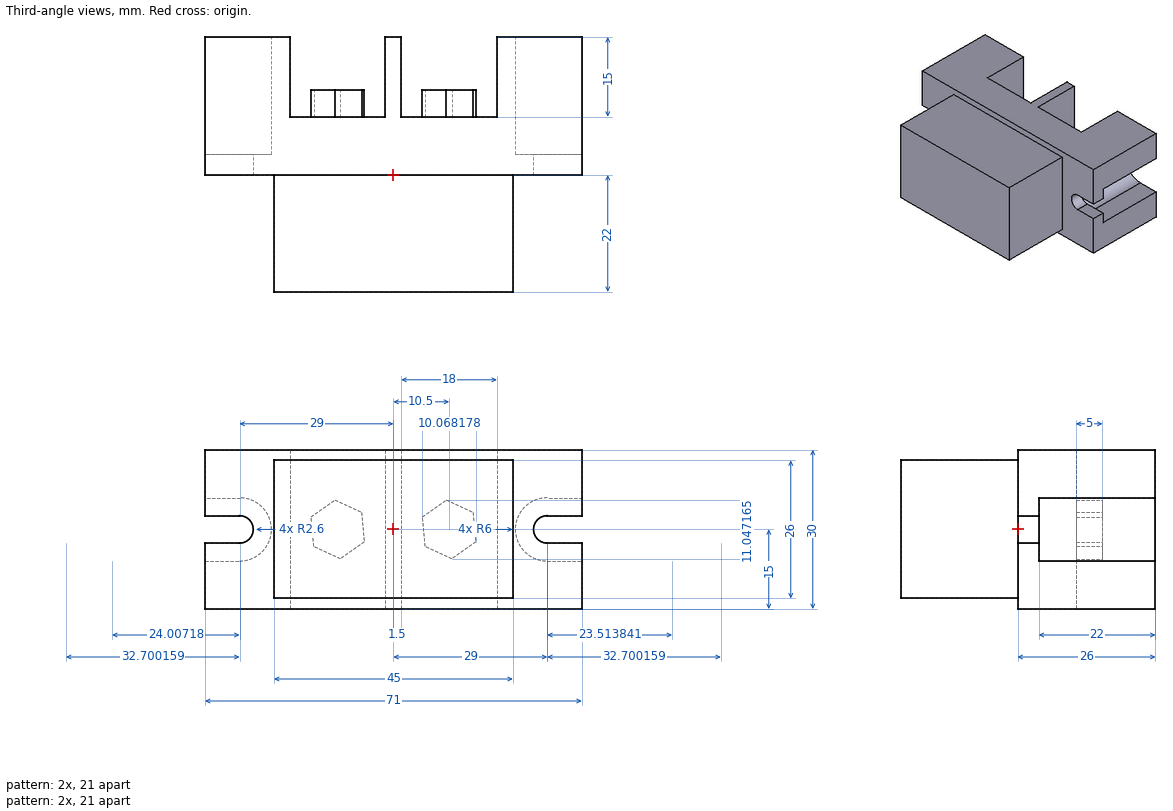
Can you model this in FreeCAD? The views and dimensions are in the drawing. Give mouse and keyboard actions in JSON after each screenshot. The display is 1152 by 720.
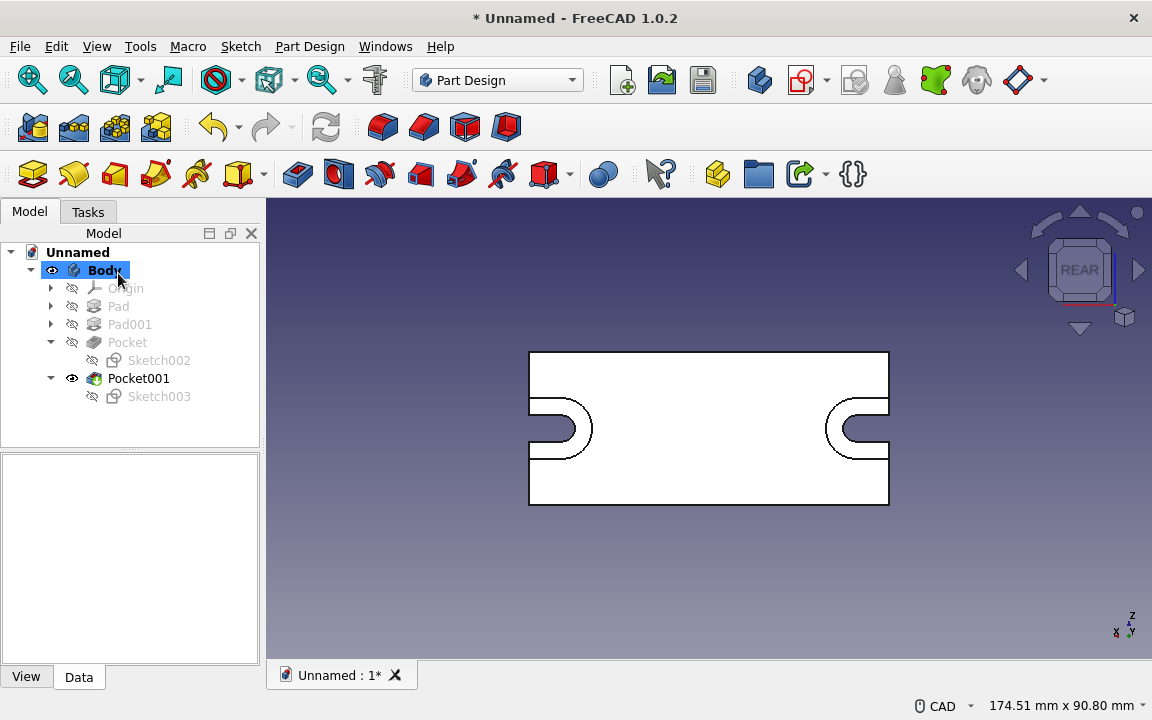
{"action": "left_click", "coordinate": [33, 80]}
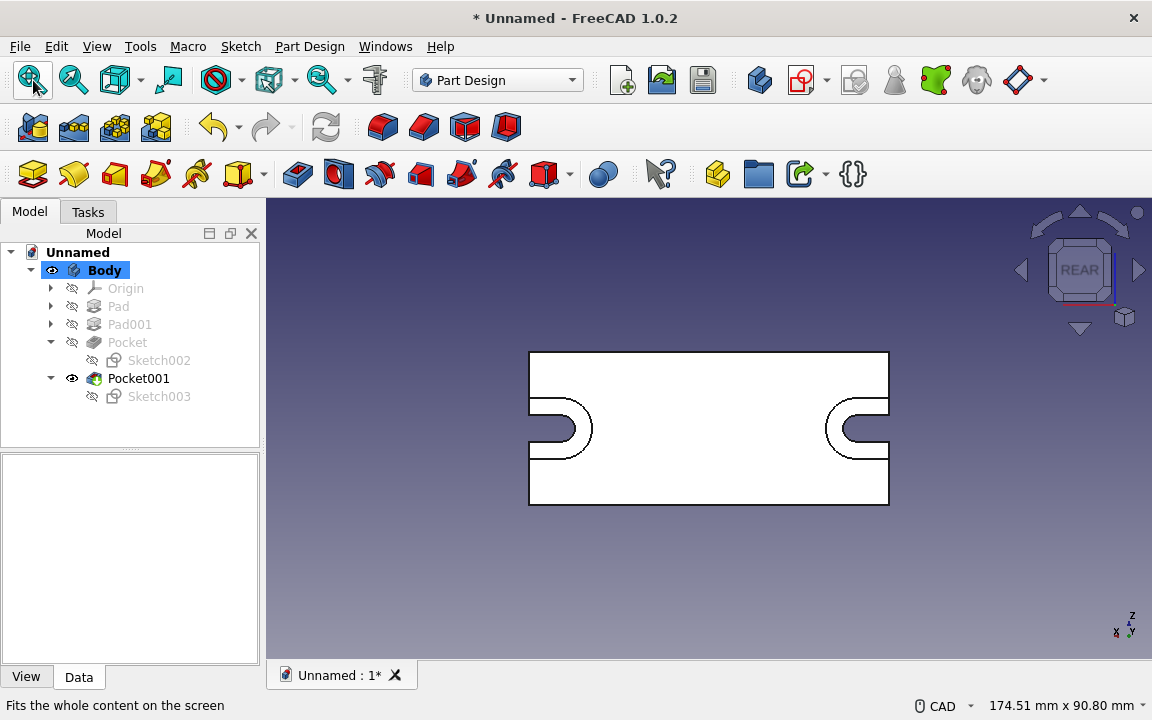
{"action": "left_click", "coordinate": [709, 427]}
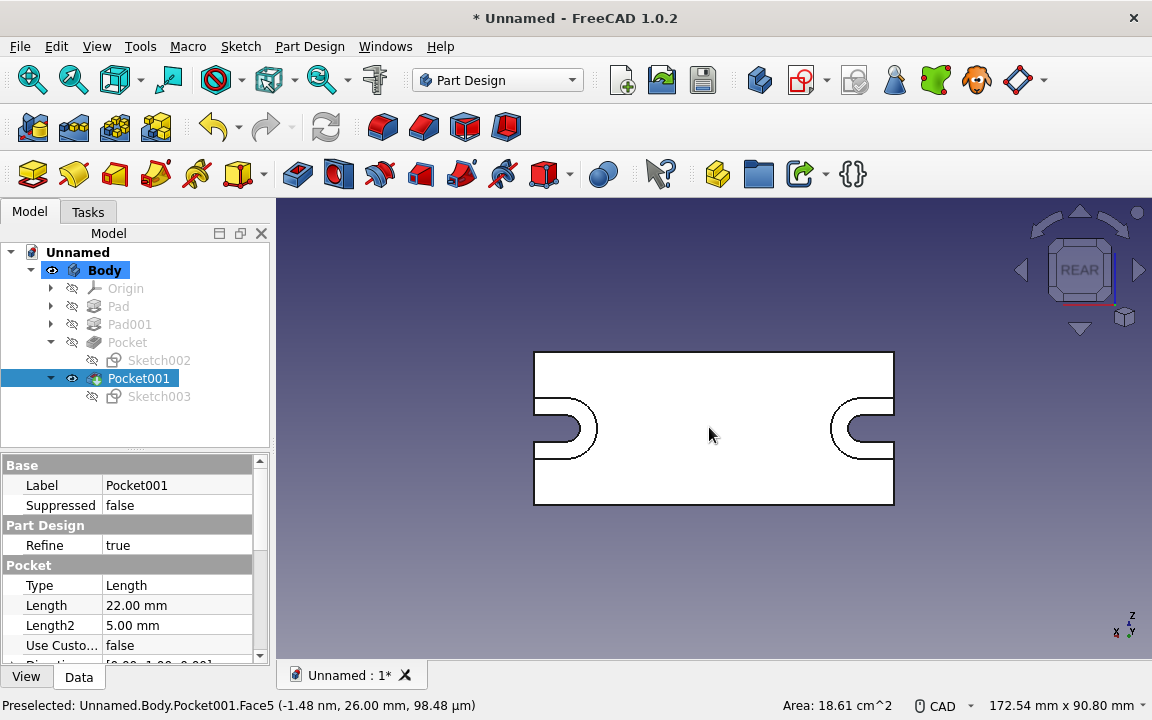
{"action": "left_click", "coordinate": [800, 80]}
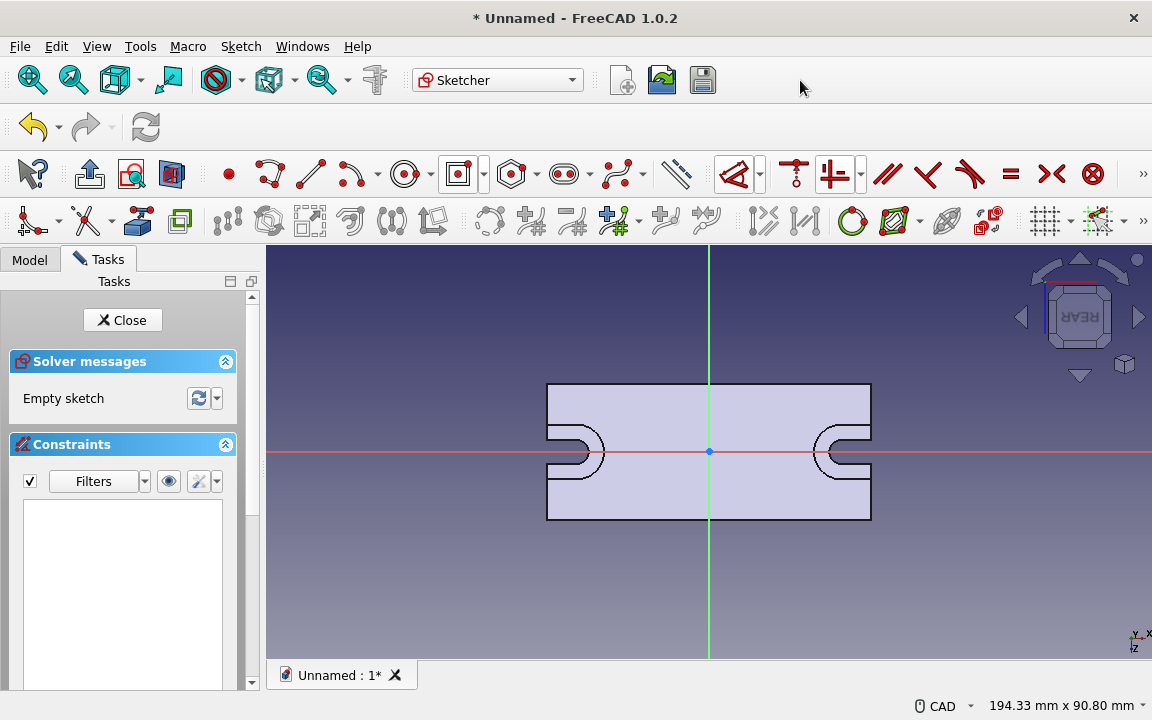
{"action": "scroll", "coordinate": [891, 452], "scroll_direction": "up", "scroll_amount": 3}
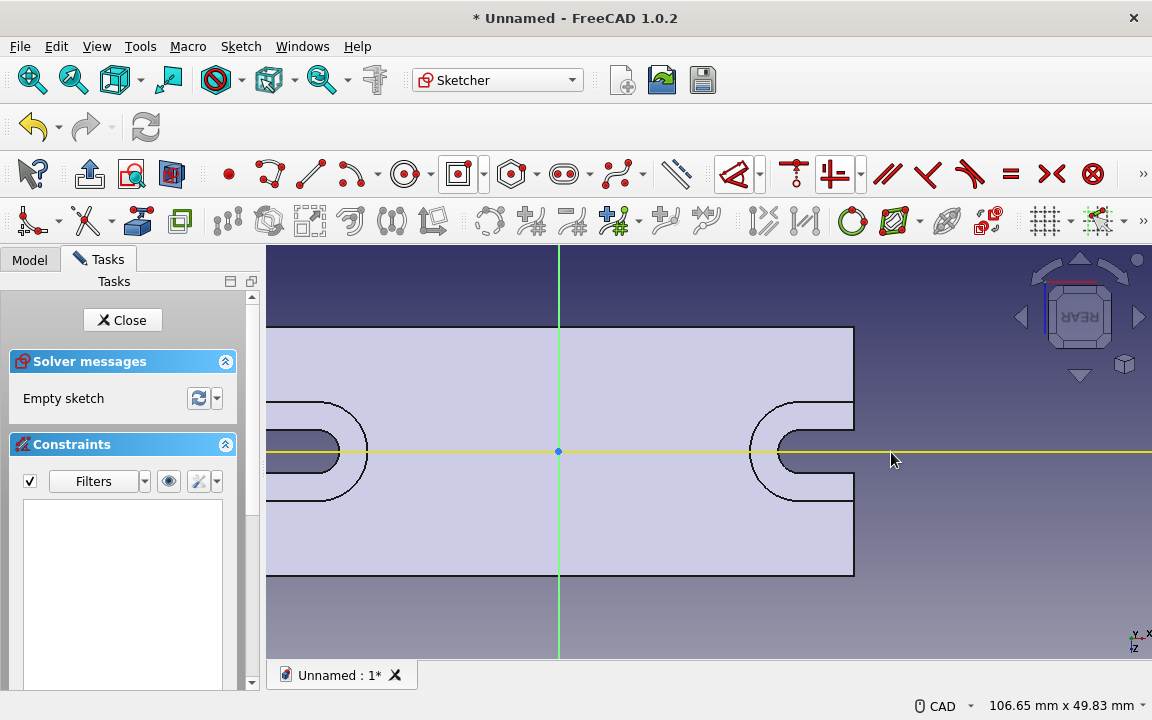
{"action": "key", "text": "g r"}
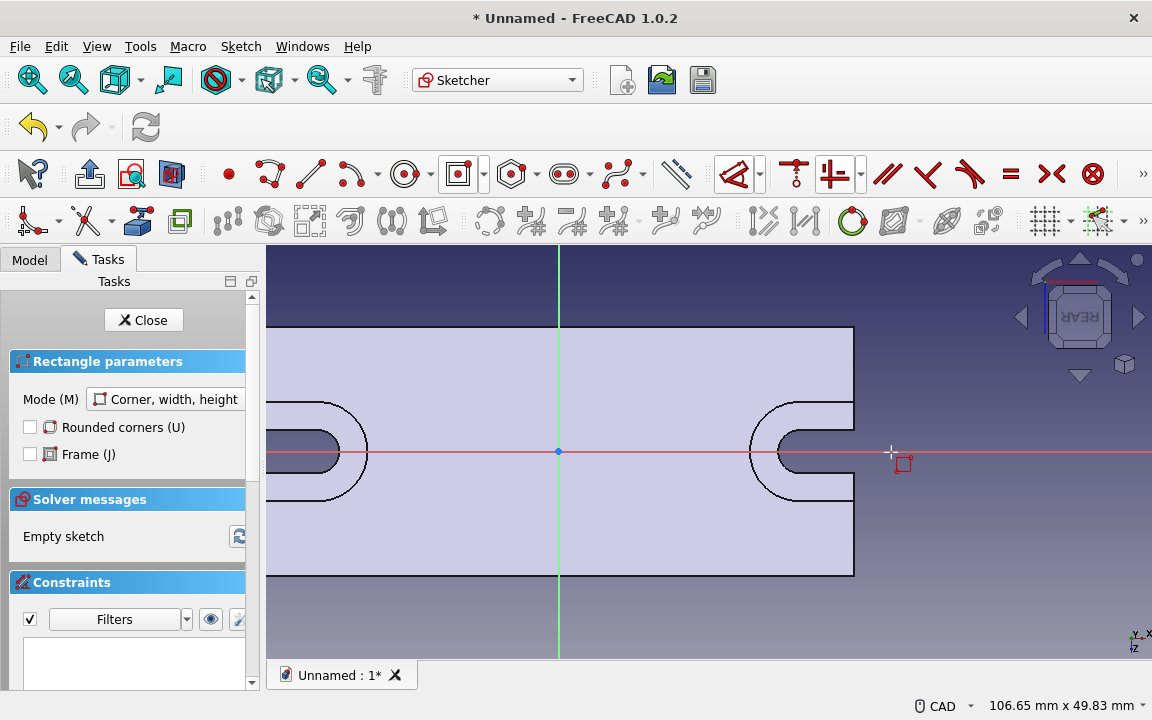
{"action": "scroll", "coordinate": [571, 327], "scroll_direction": "up", "scroll_amount": 2}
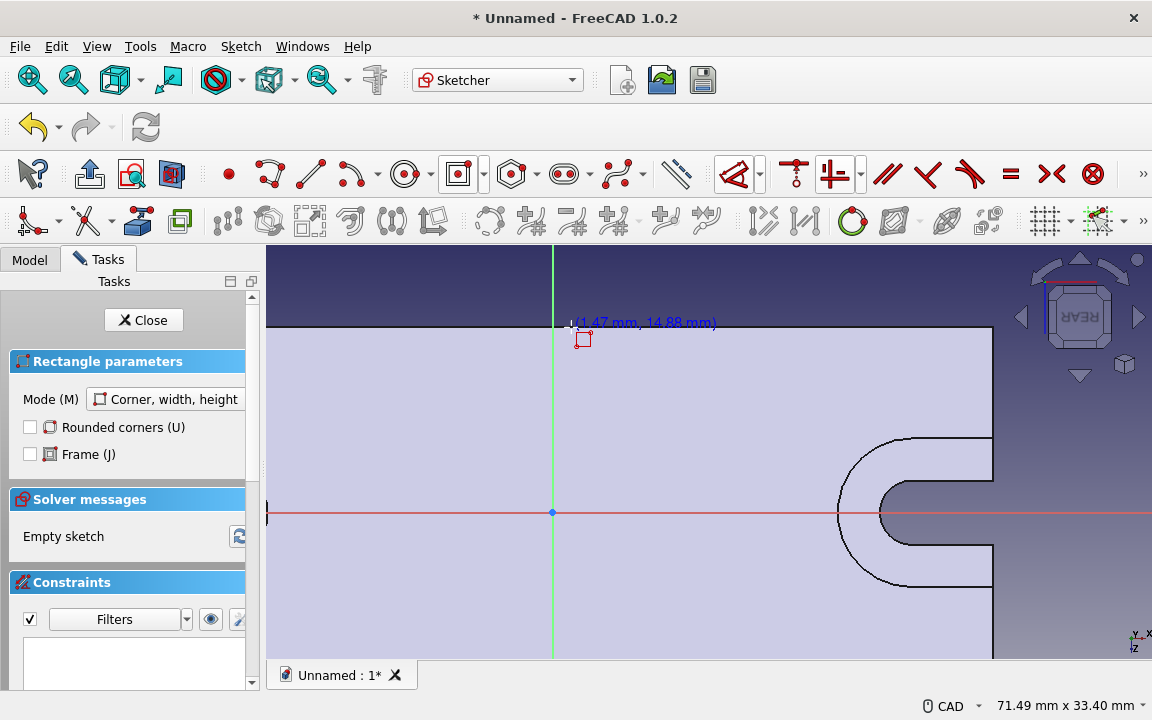
{"action": "left_click", "coordinate": [571, 327]}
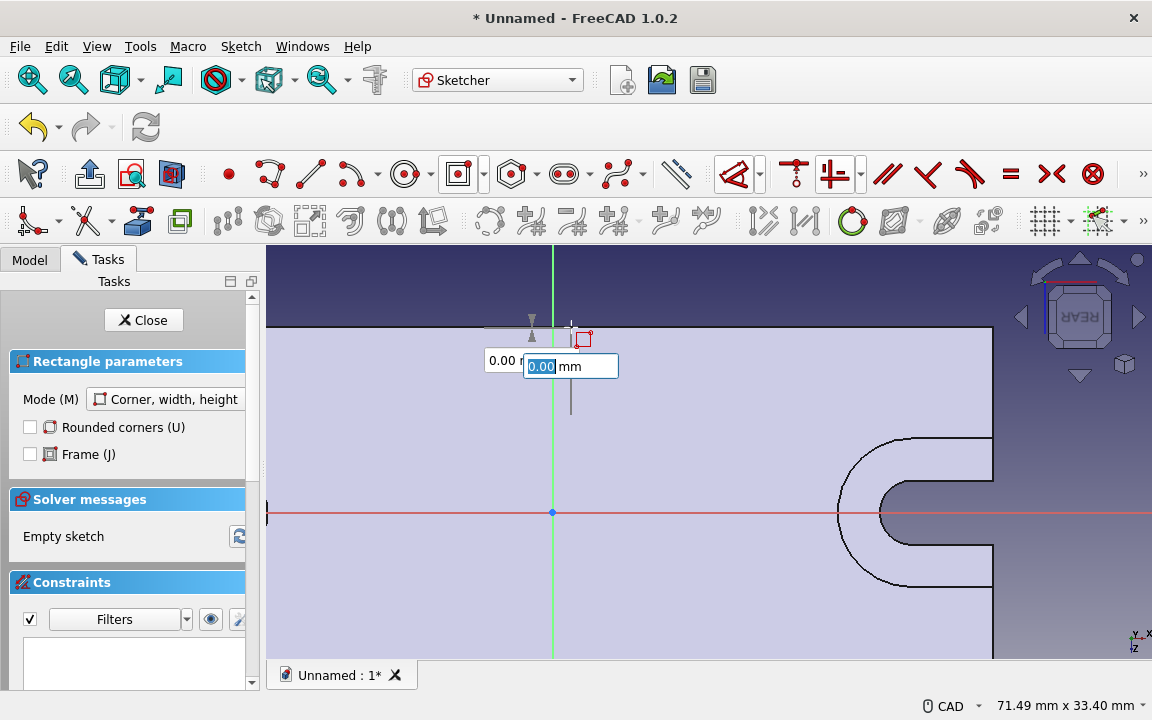
{"action": "scroll", "coordinate": [573, 328], "scroll_direction": "down", "scroll_amount": 2}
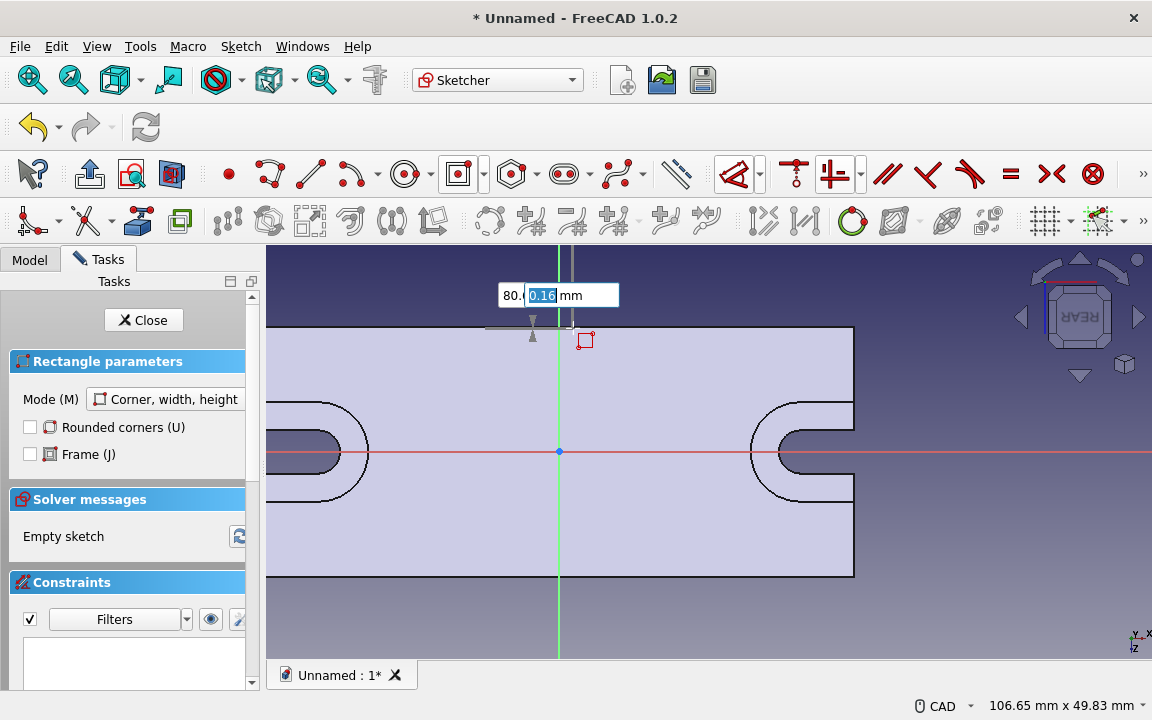
{"action": "left_click", "coordinate": [721, 577]}
{"action": "key", "text": "Escape"}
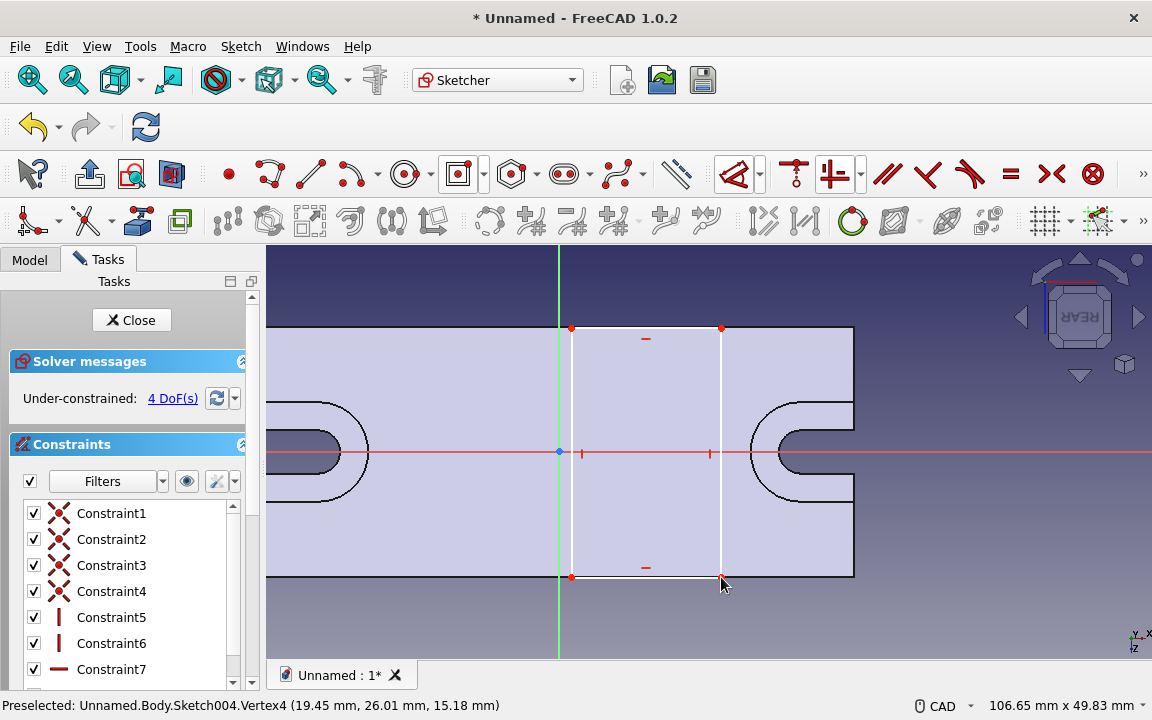
{"action": "left_click", "coordinate": [572, 403]}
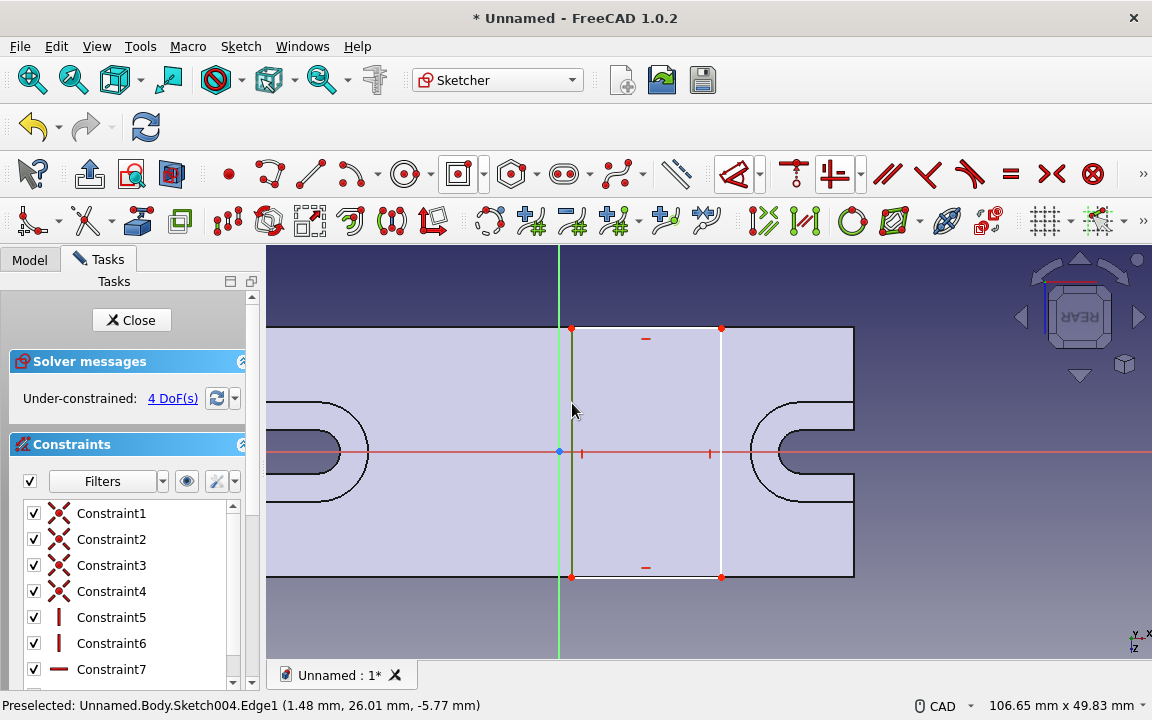
{"action": "left_click", "coordinate": [760, 174]}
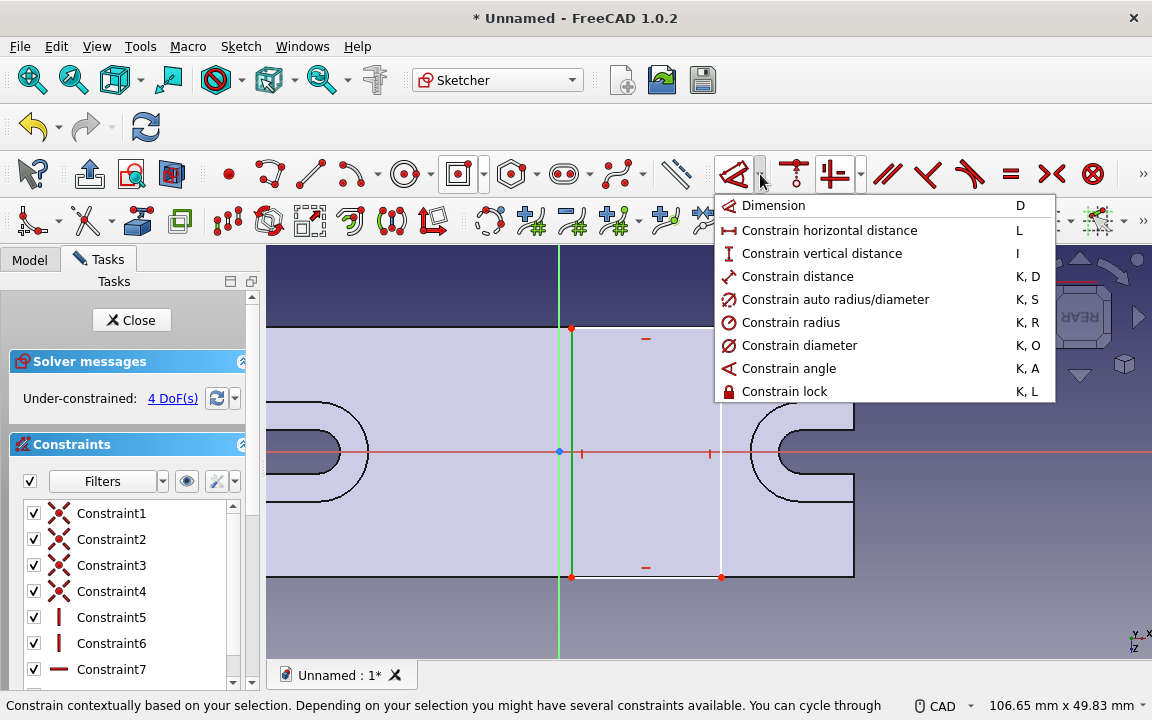
{"action": "left_click", "coordinate": [885, 254]}